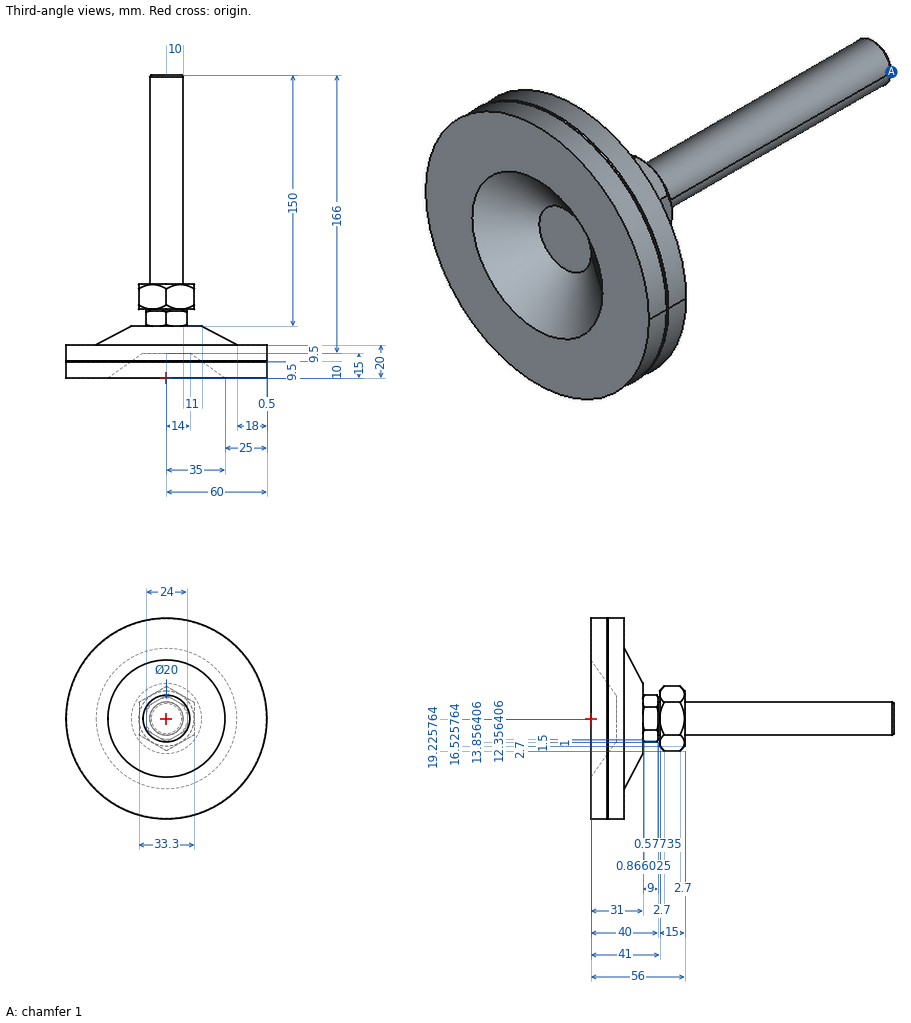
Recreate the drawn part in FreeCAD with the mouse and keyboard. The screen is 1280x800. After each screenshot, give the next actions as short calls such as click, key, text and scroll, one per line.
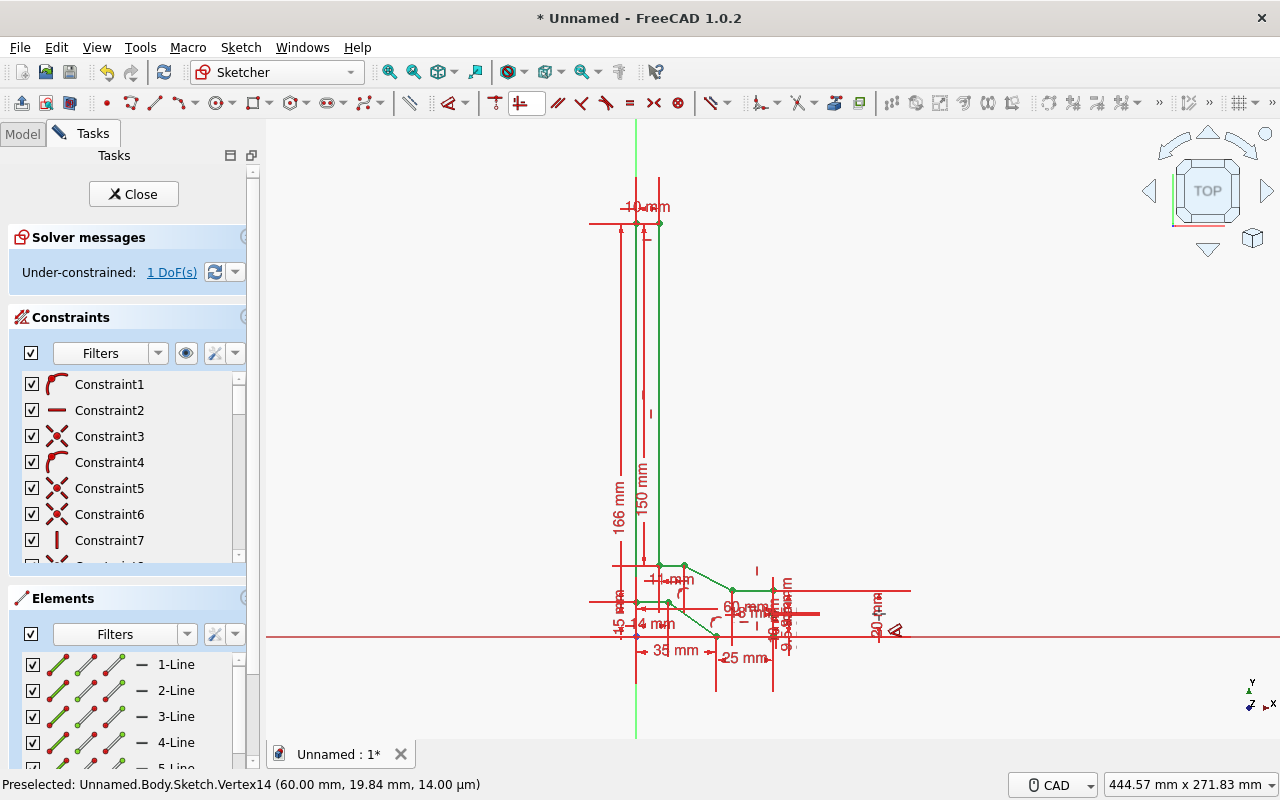
scroll(773, 614, up, 18)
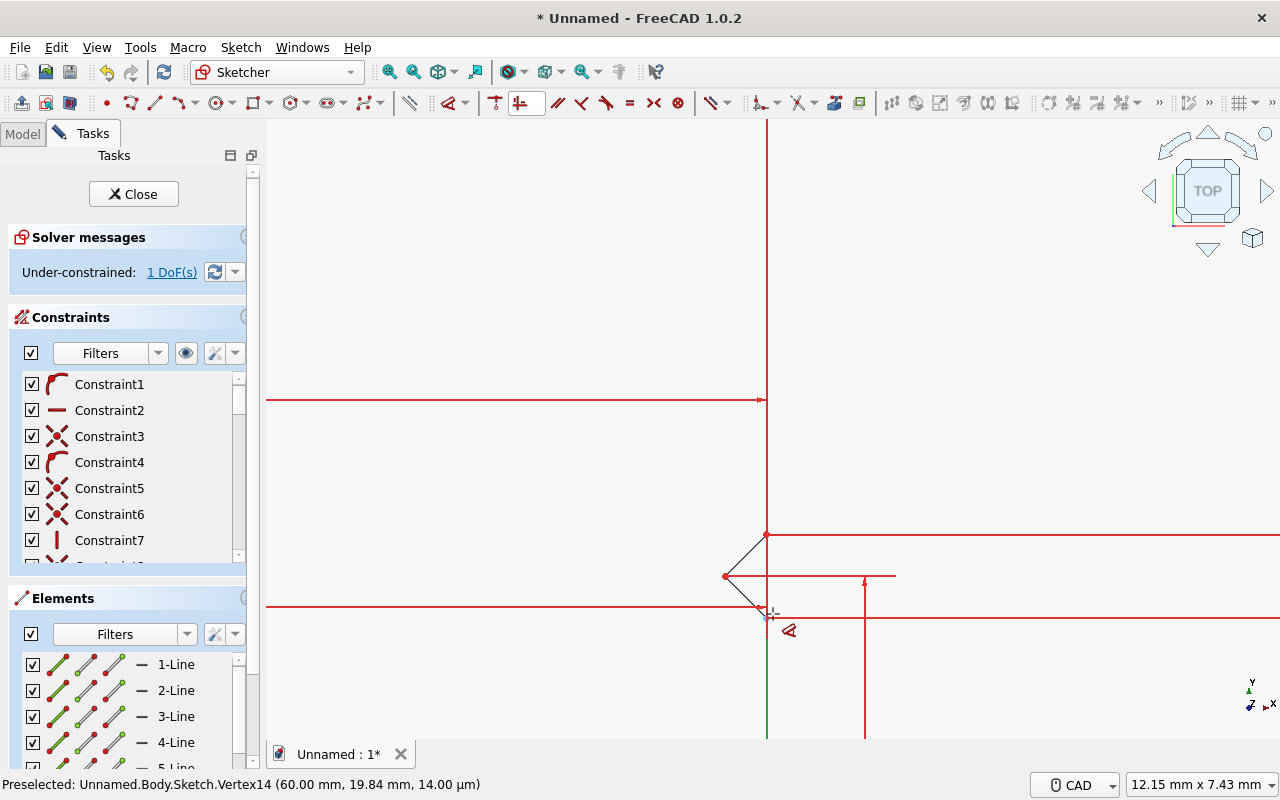
click(746, 597)
click(746, 652)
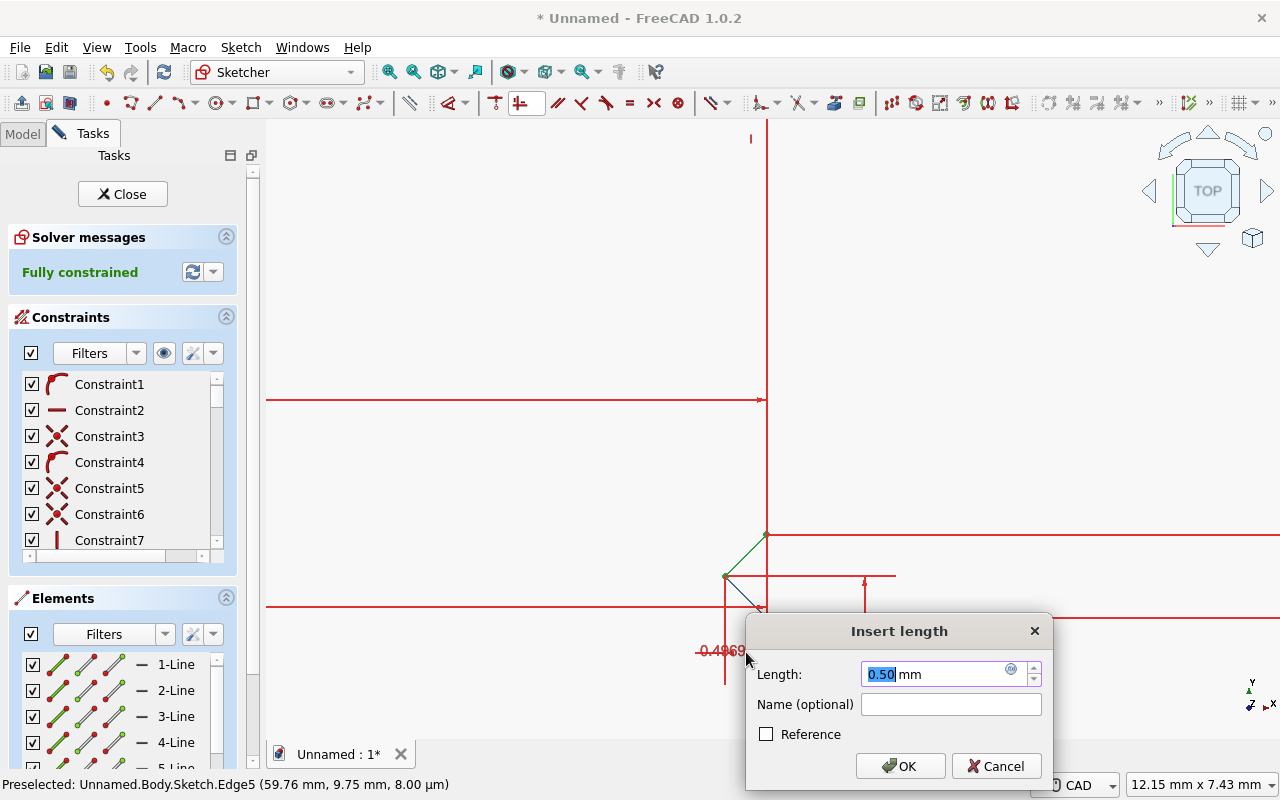
text(0.5)
key(Return)
key(Escape)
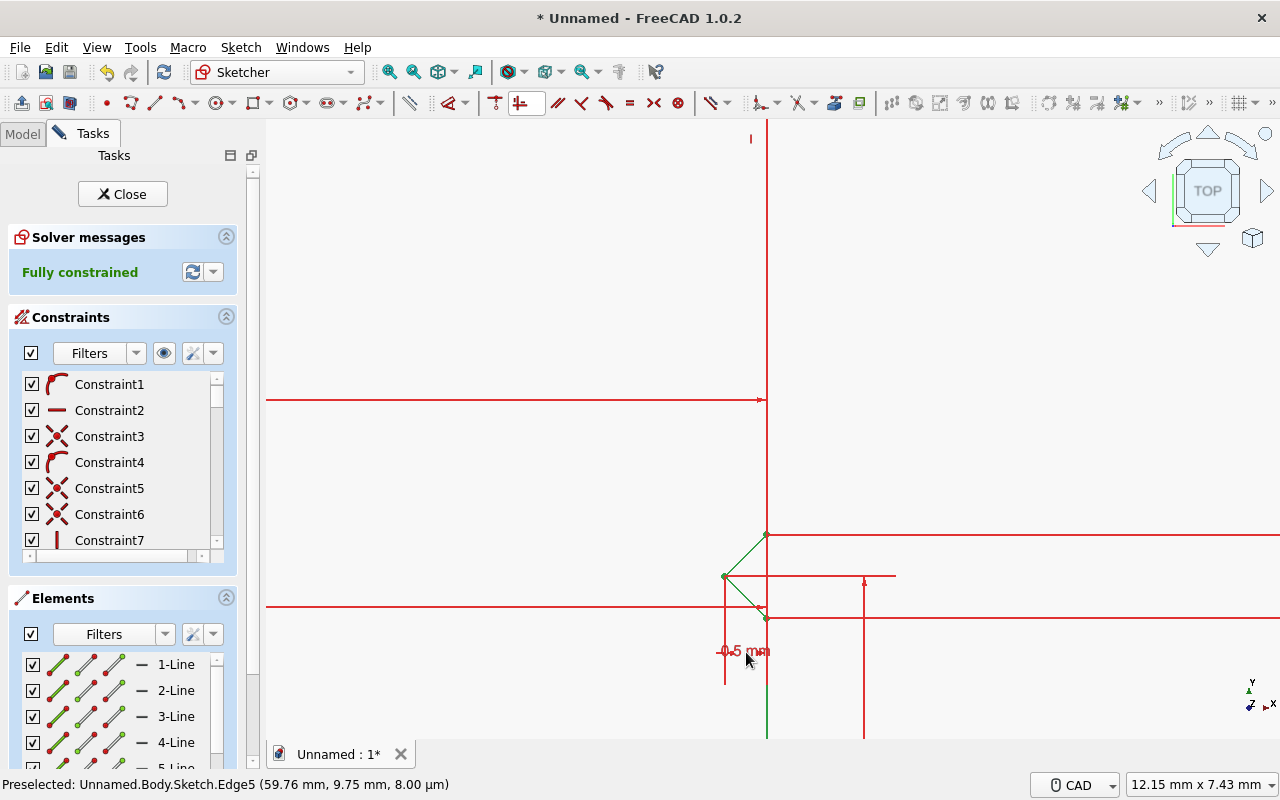
click(123, 194)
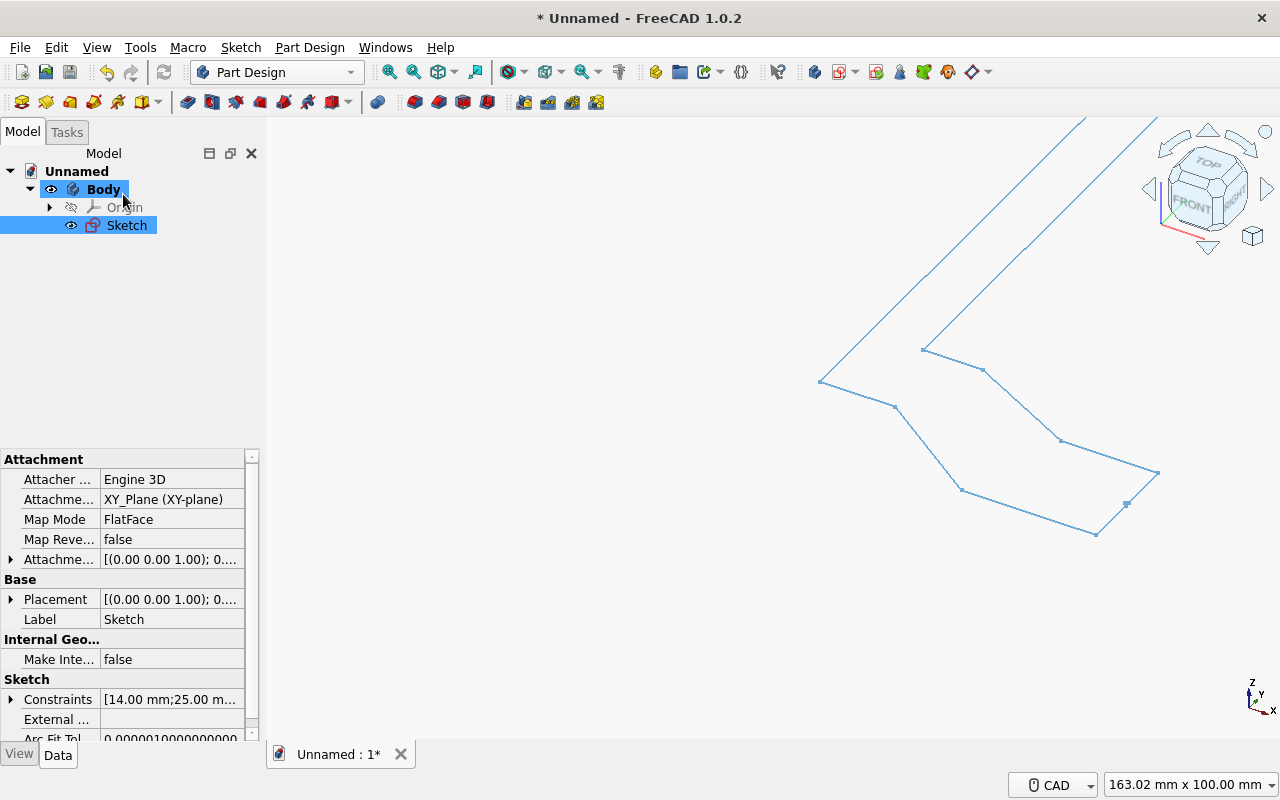
click(46, 102)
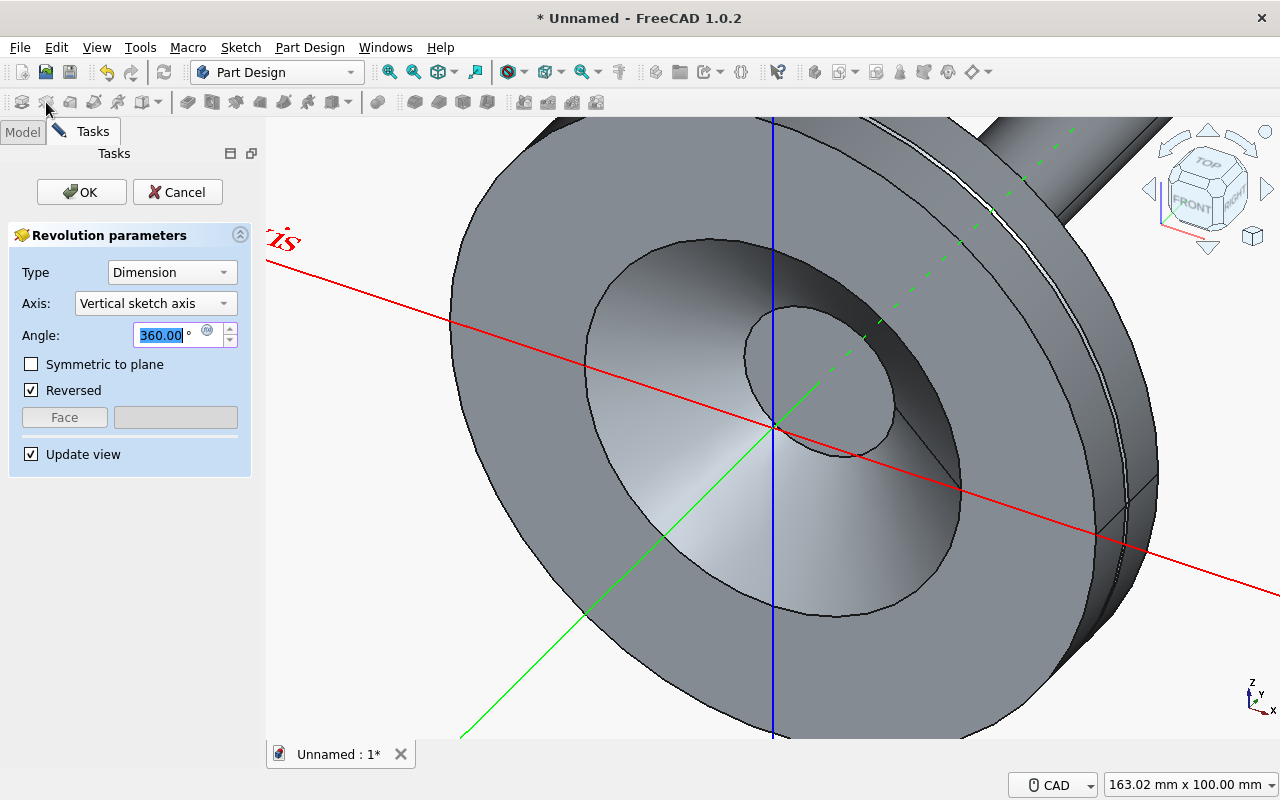
click(82, 192)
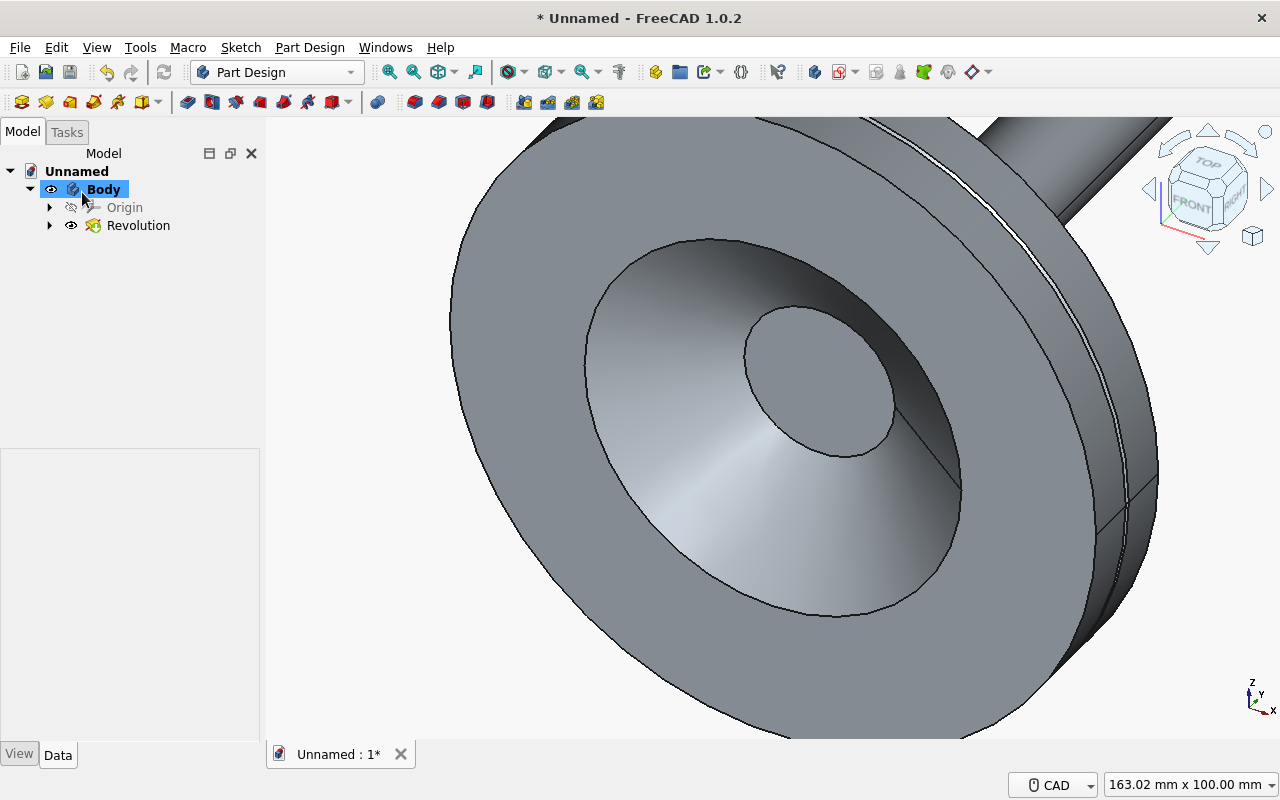
click(390, 72)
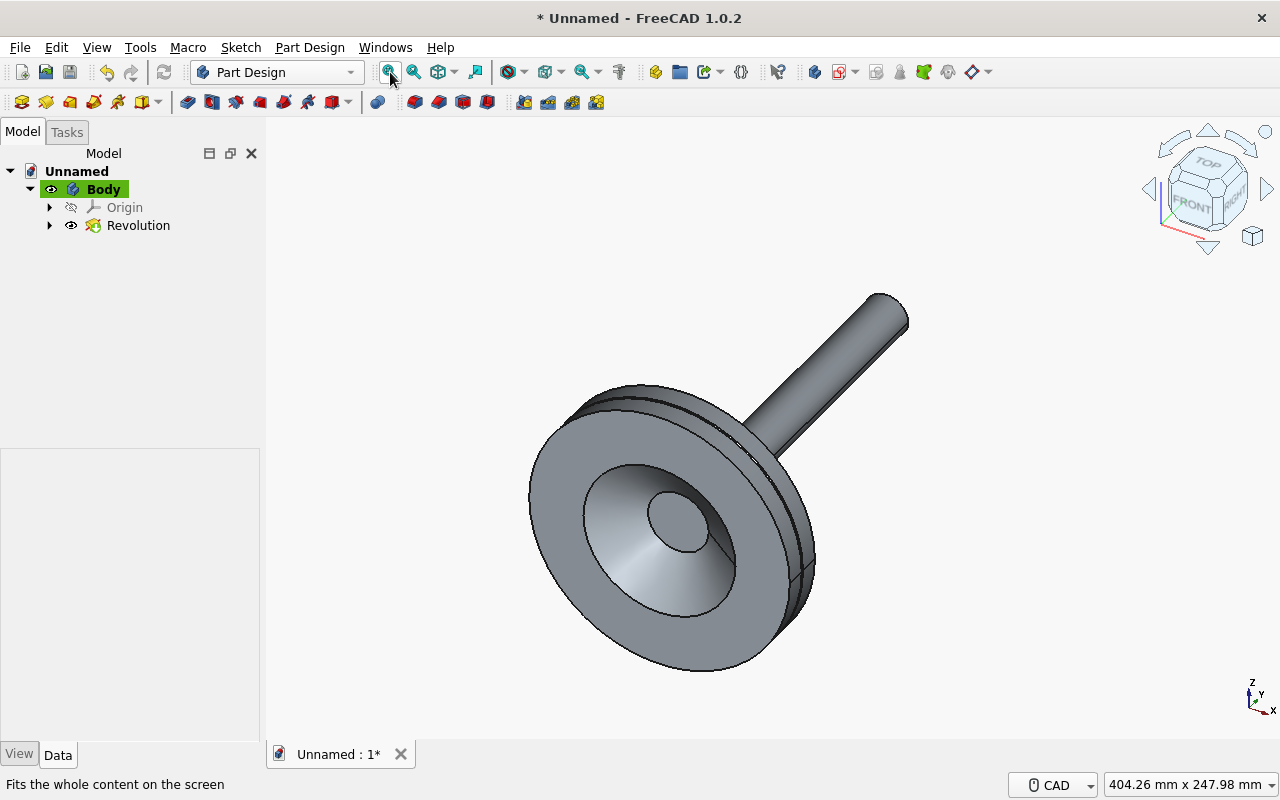
key(4)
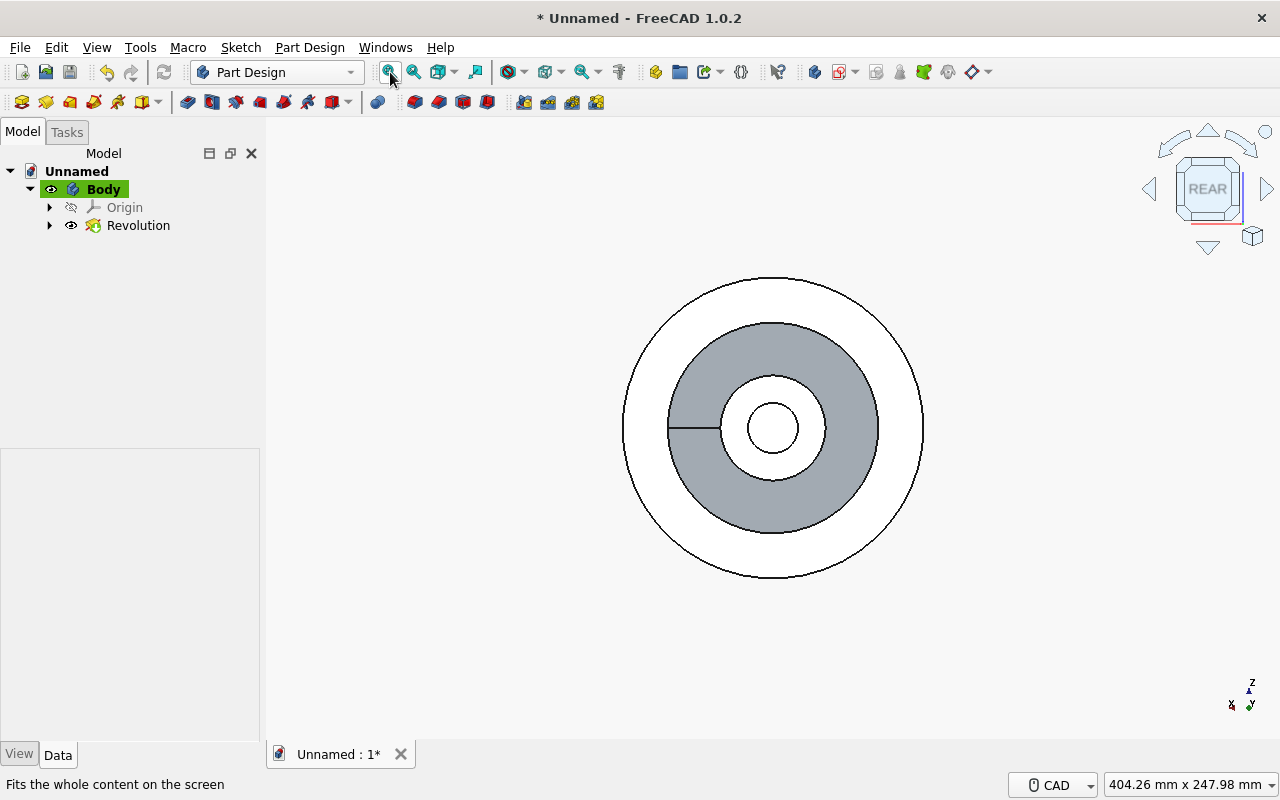
click(803, 457)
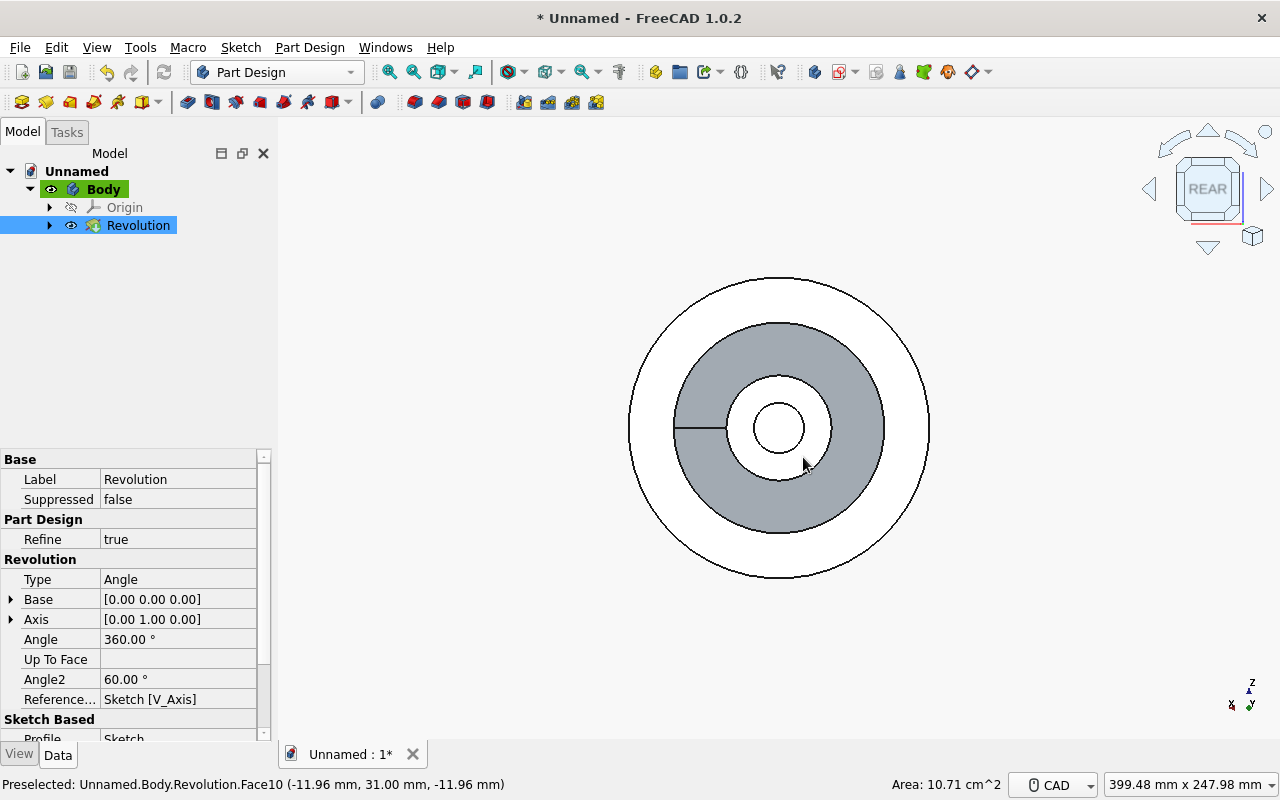
click(840, 72)